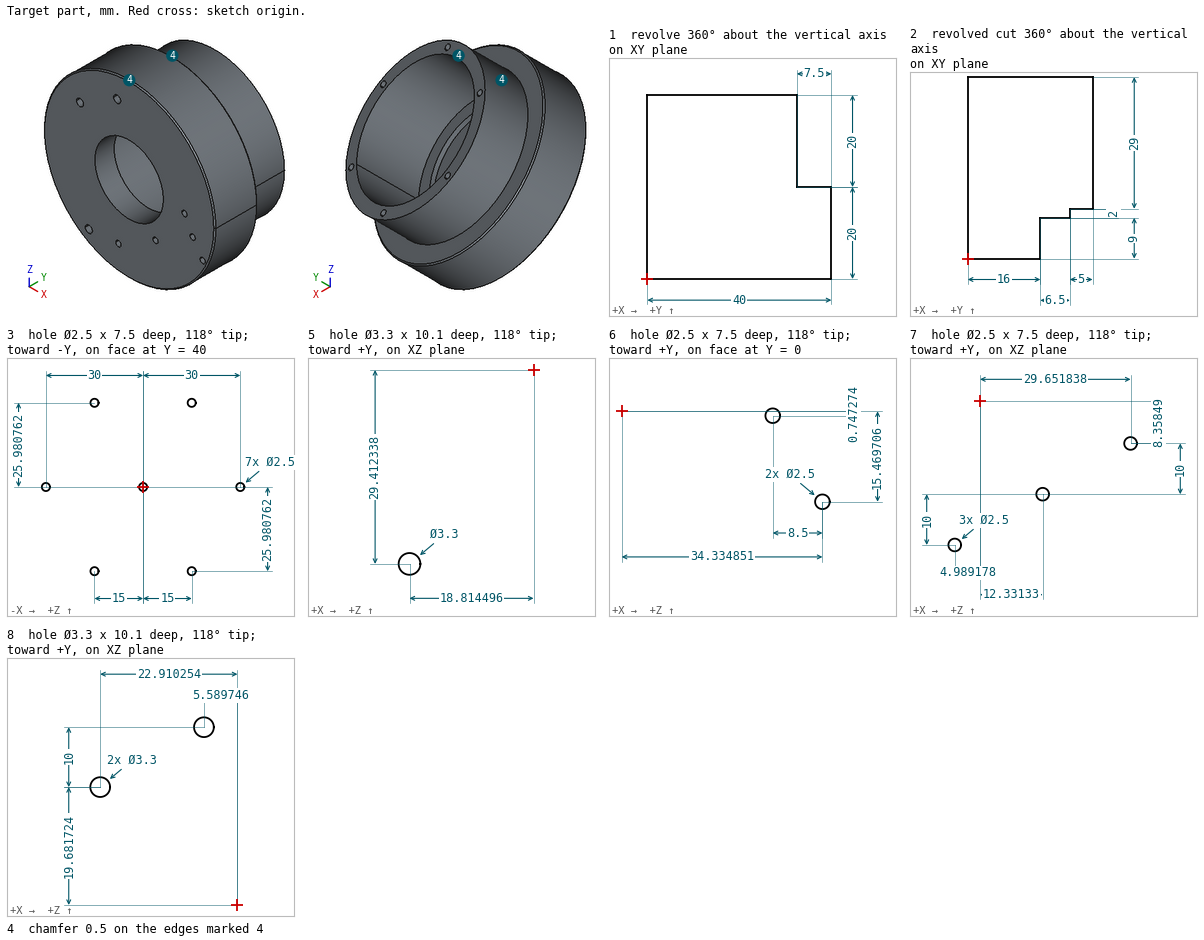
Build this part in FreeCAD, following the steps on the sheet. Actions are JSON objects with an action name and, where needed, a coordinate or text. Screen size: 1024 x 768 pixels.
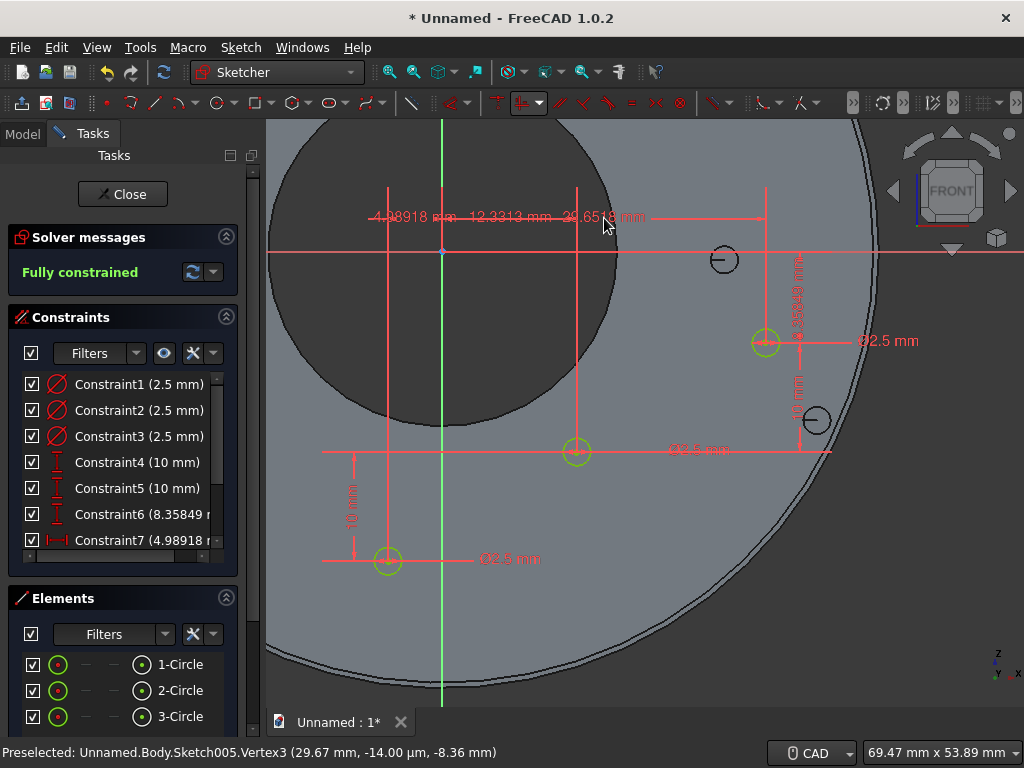
{"action": "left_click", "coordinate": [123, 194]}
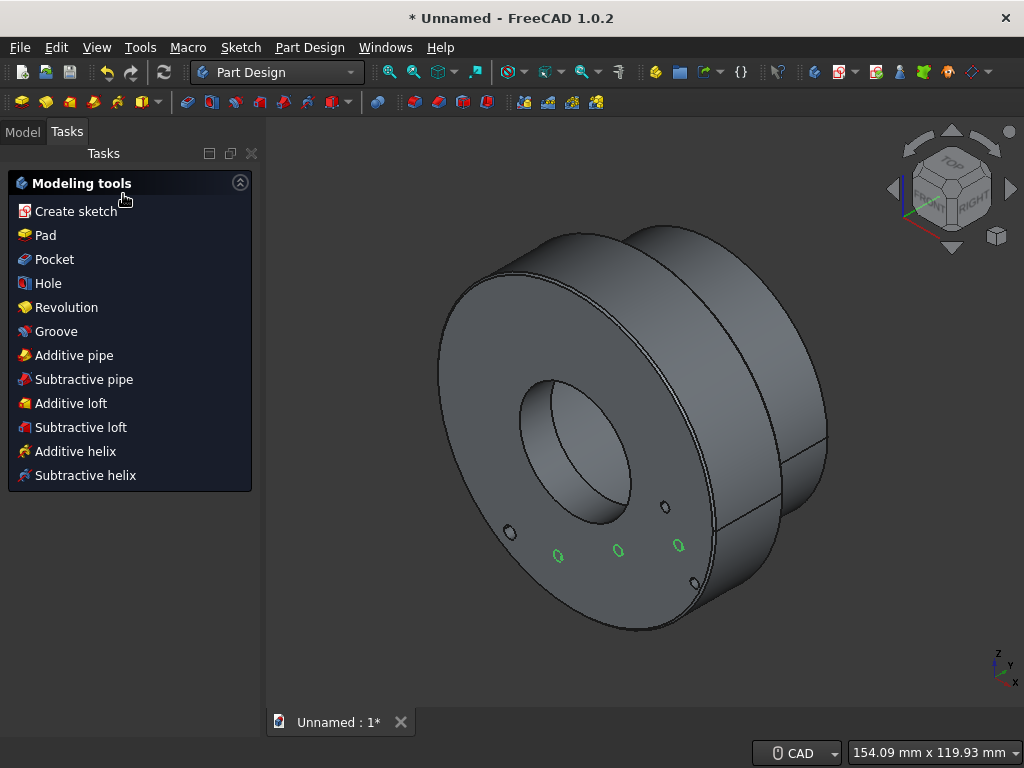
{"action": "left_click", "coordinate": [212, 102]}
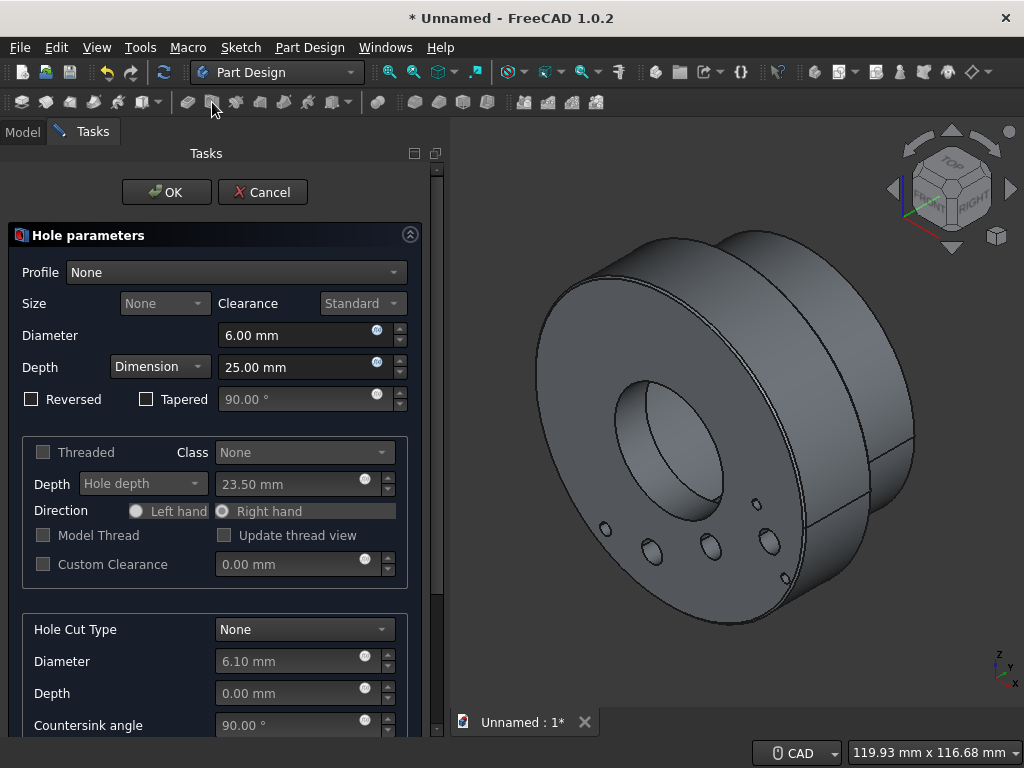
{"action": "triple_click", "coordinate": [305, 335]}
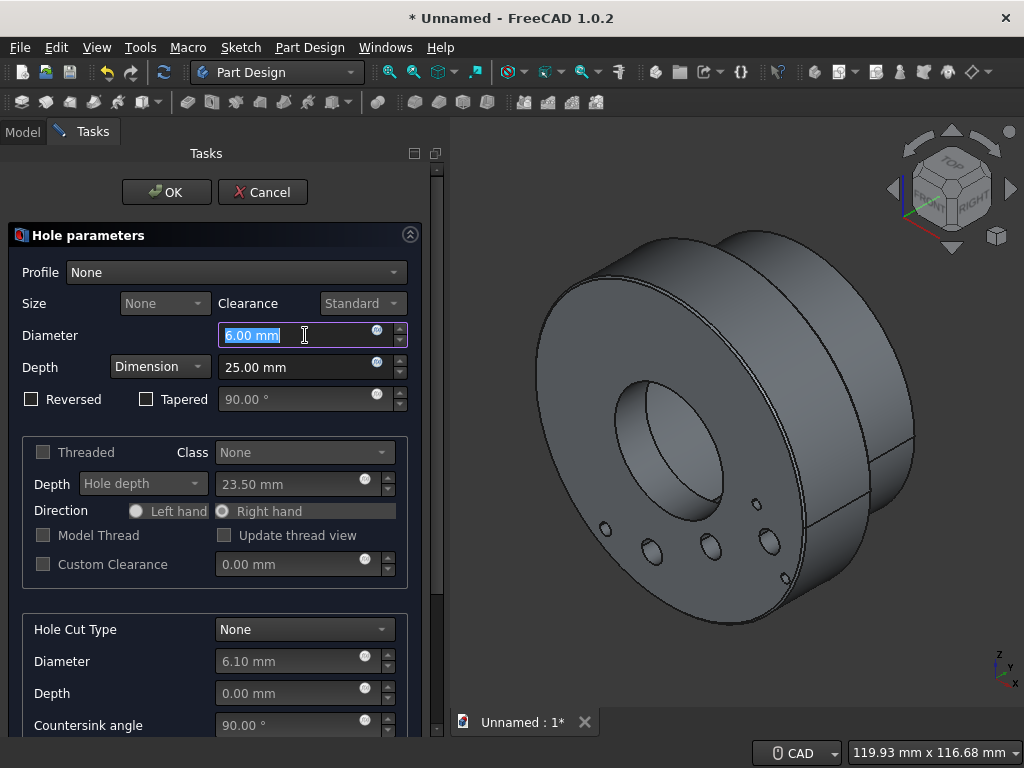
{"action": "type", "text": "2.5"}
{"action": "key", "text": "Tab"}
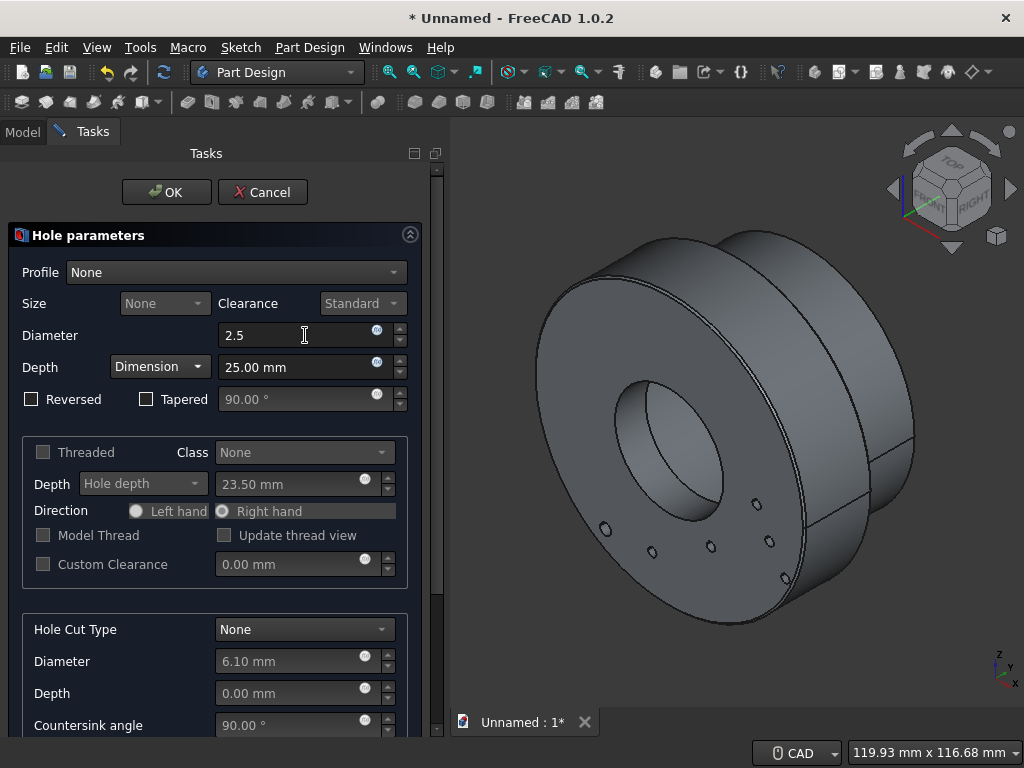
{"action": "triple_click", "coordinate": [305, 367]}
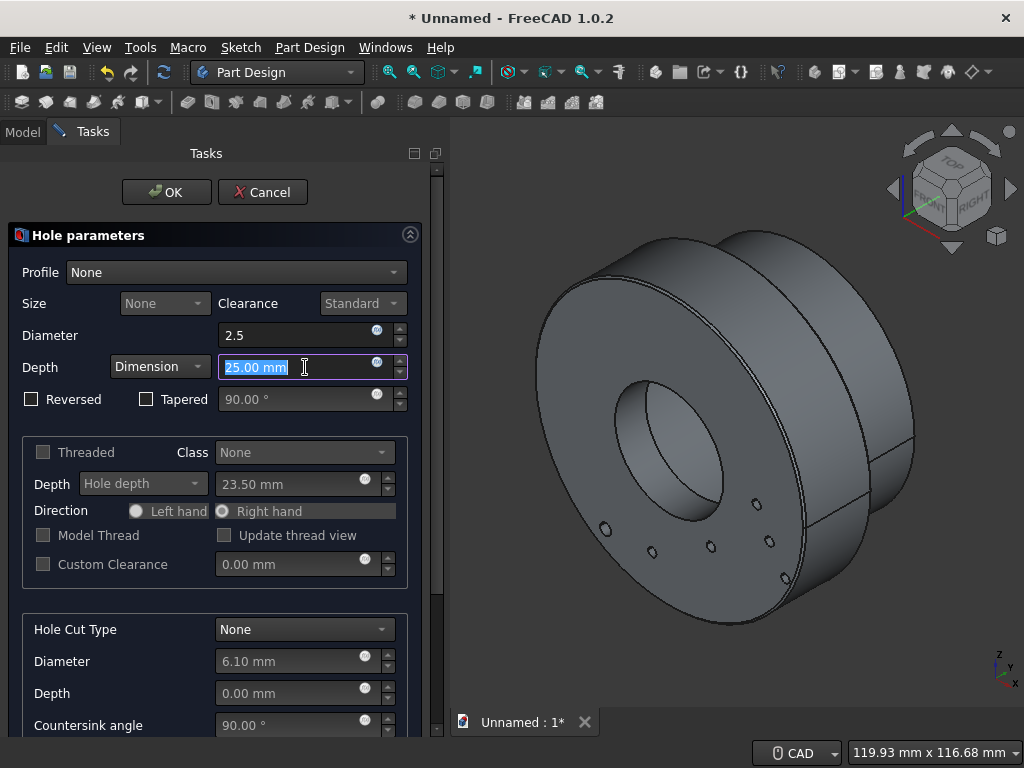
{"action": "type", "text": "7.5"}
{"action": "key", "text": "Tab"}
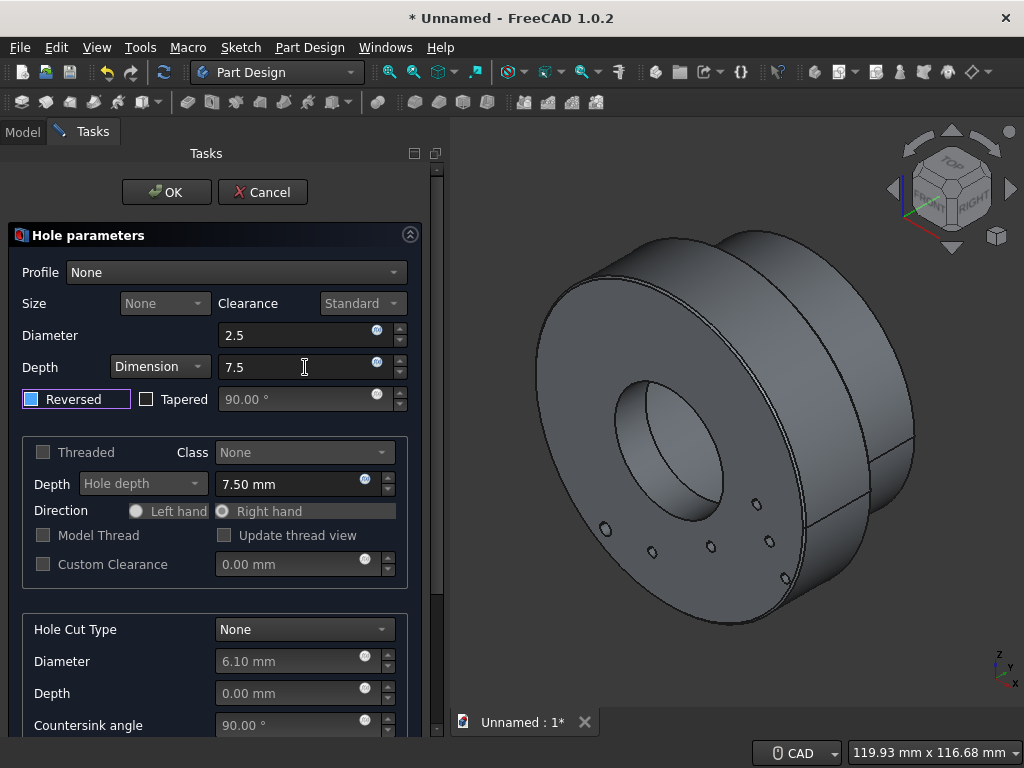
{"action": "left_click", "coordinate": [167, 192]}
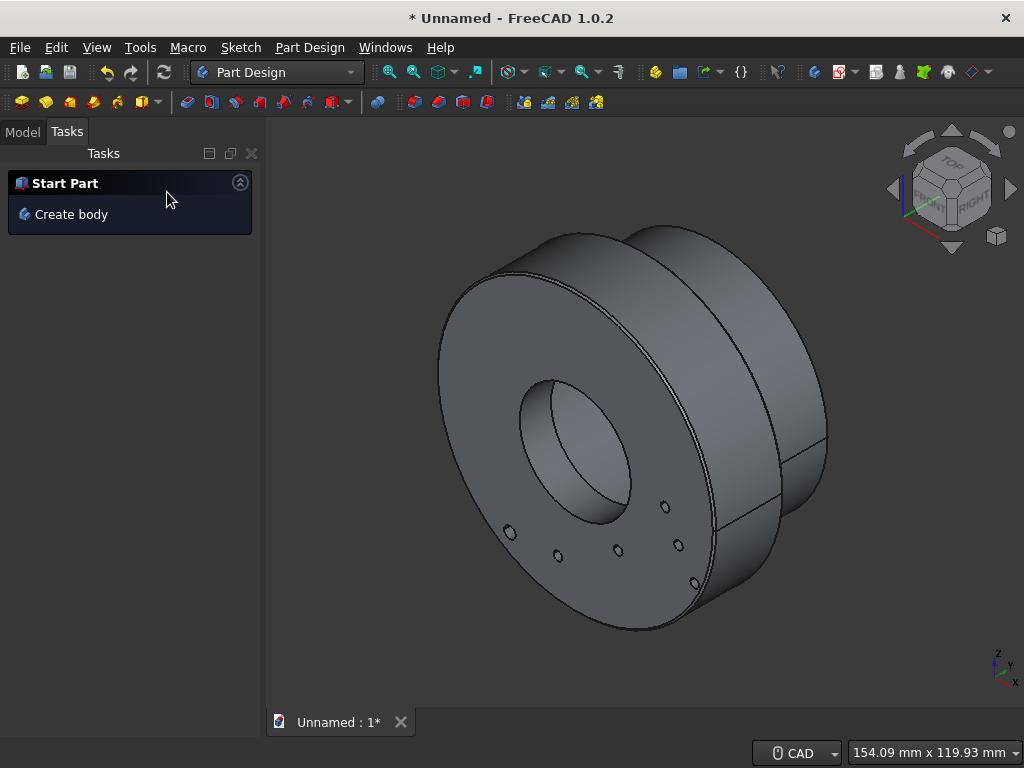
{"action": "left_click", "coordinate": [840, 72]}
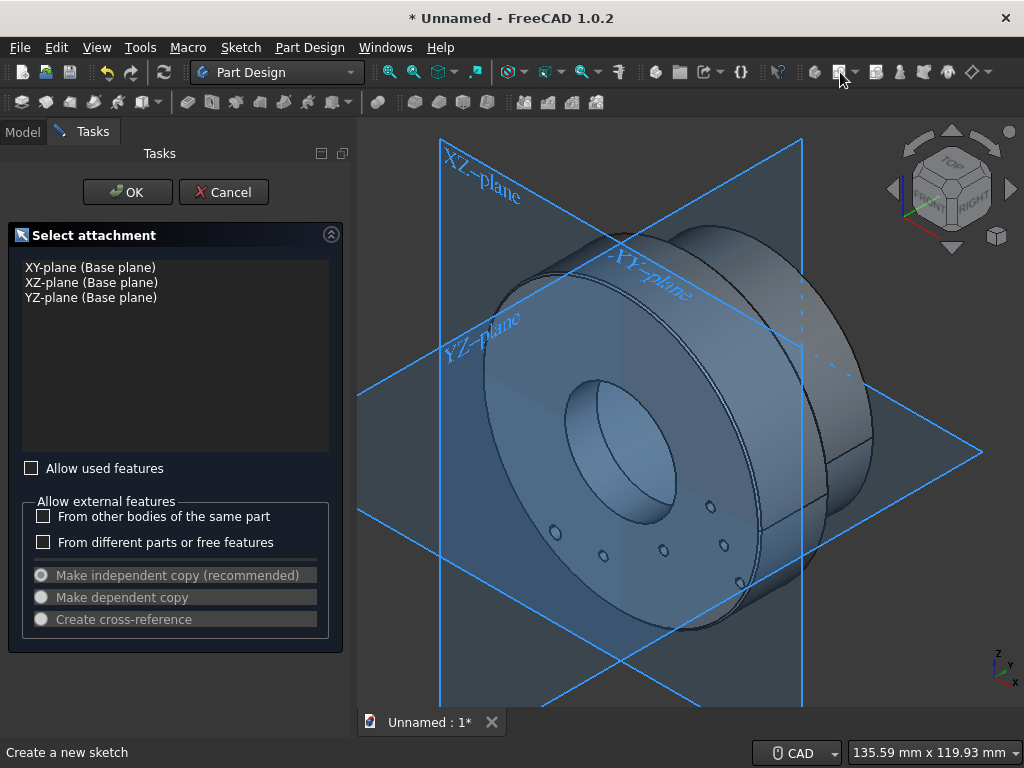
{"action": "left_click", "coordinate": [82, 282]}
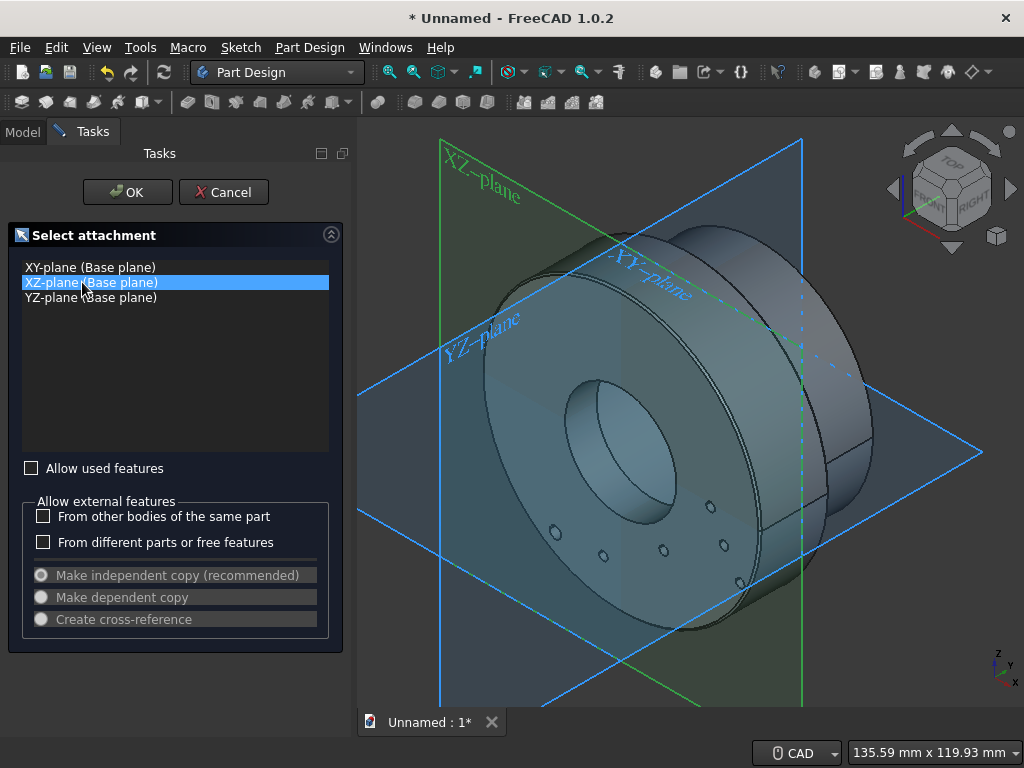
{"action": "left_click", "coordinate": [128, 192]}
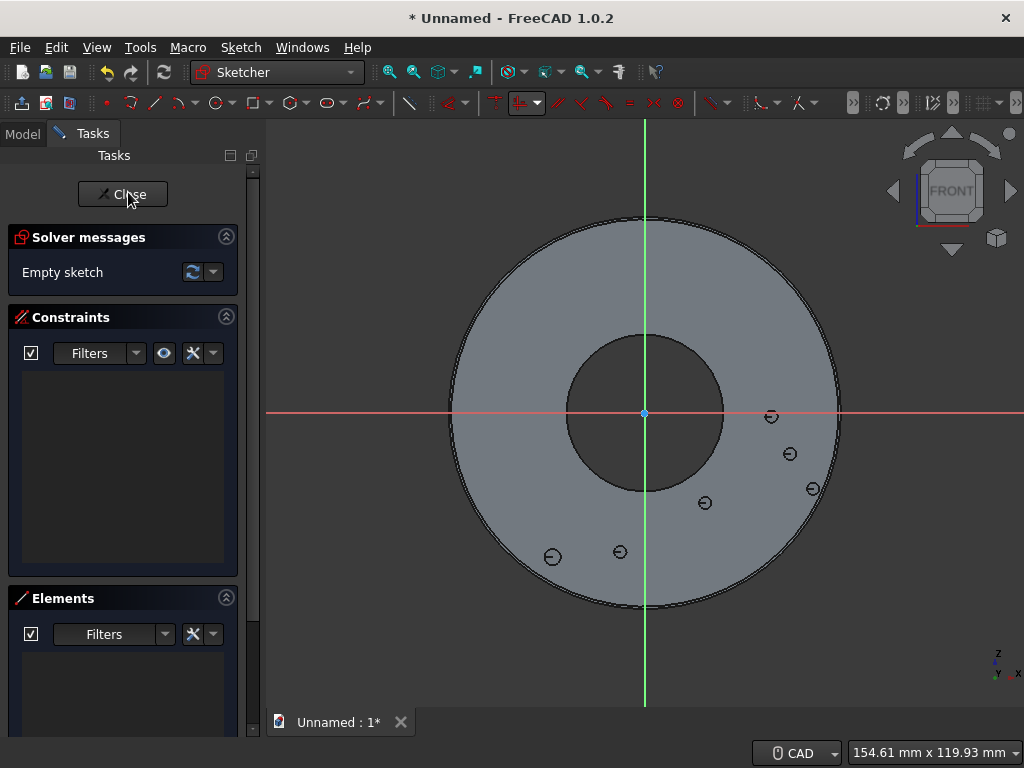
{"action": "scroll", "coordinate": [591, 274], "scroll_direction": "up", "scroll_amount": 4}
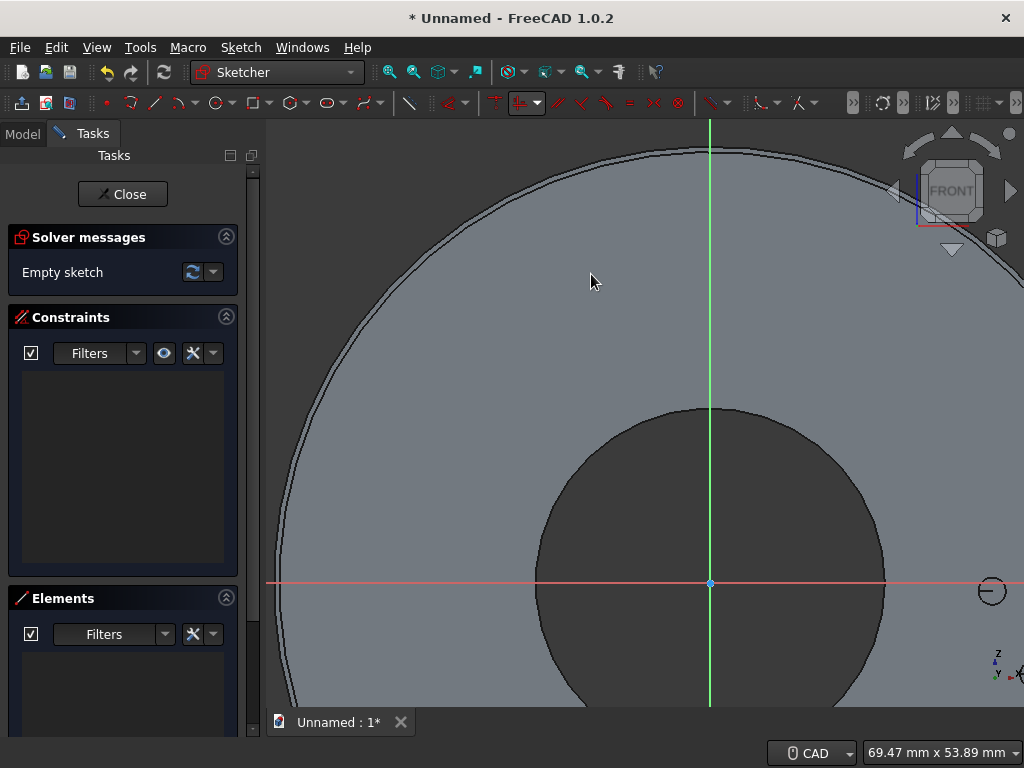
{"action": "left_click", "coordinate": [216, 104]}